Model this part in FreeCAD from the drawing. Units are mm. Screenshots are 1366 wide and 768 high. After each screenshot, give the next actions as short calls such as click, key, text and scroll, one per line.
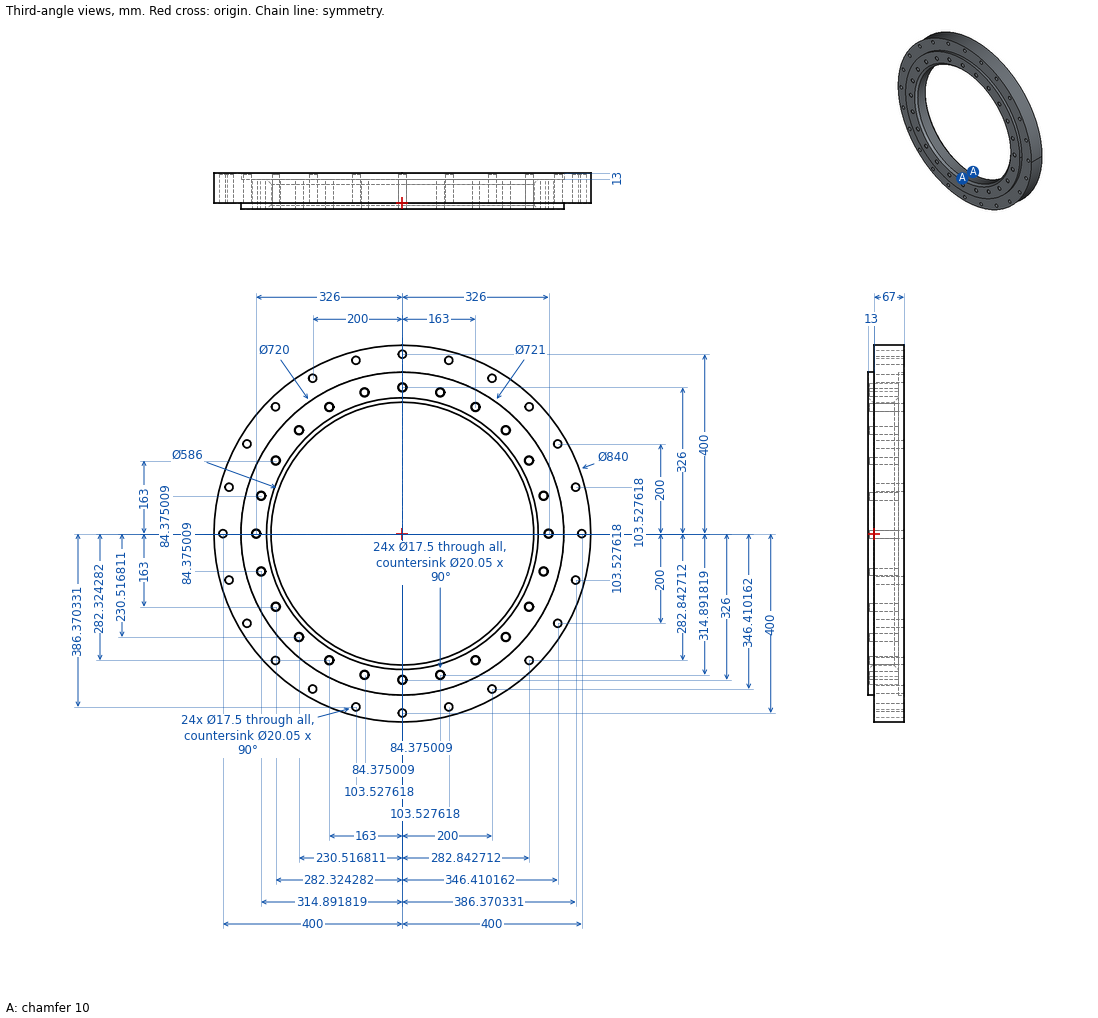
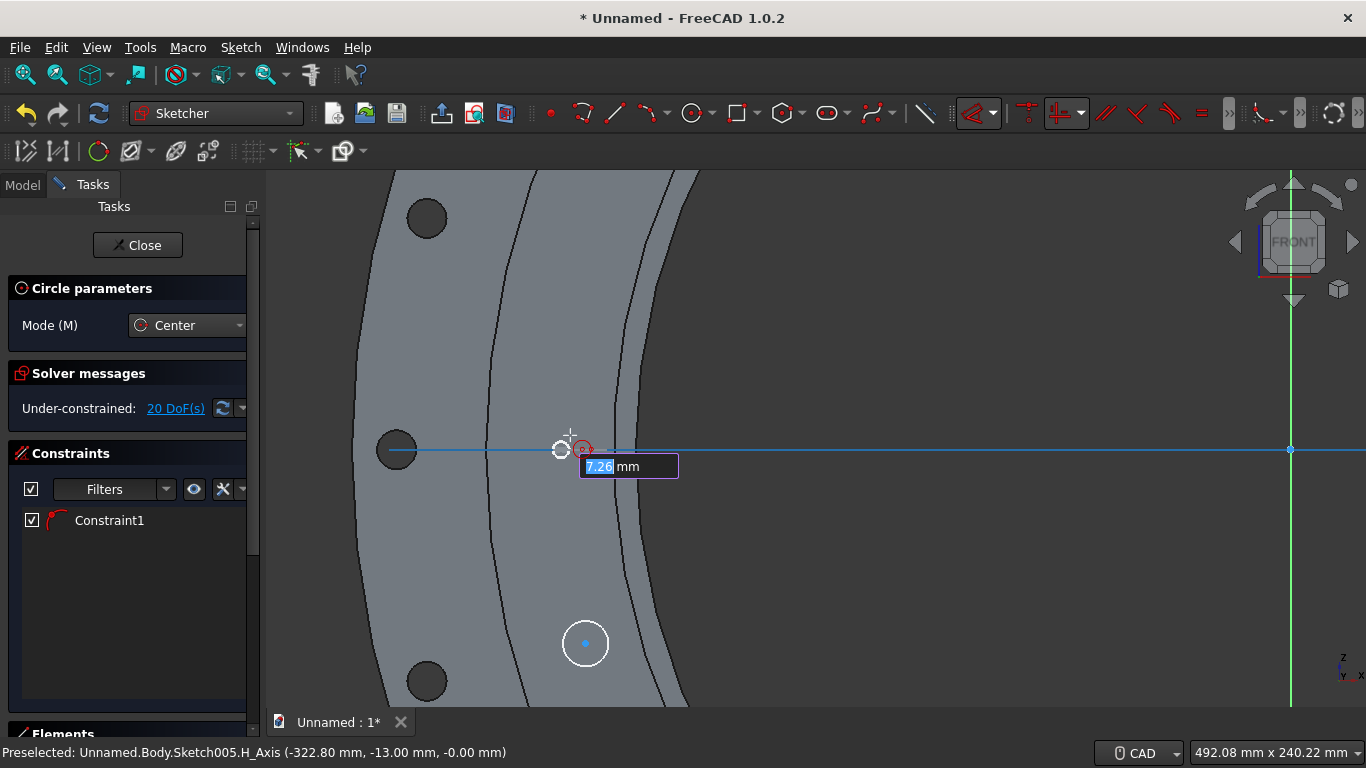
click(569, 431)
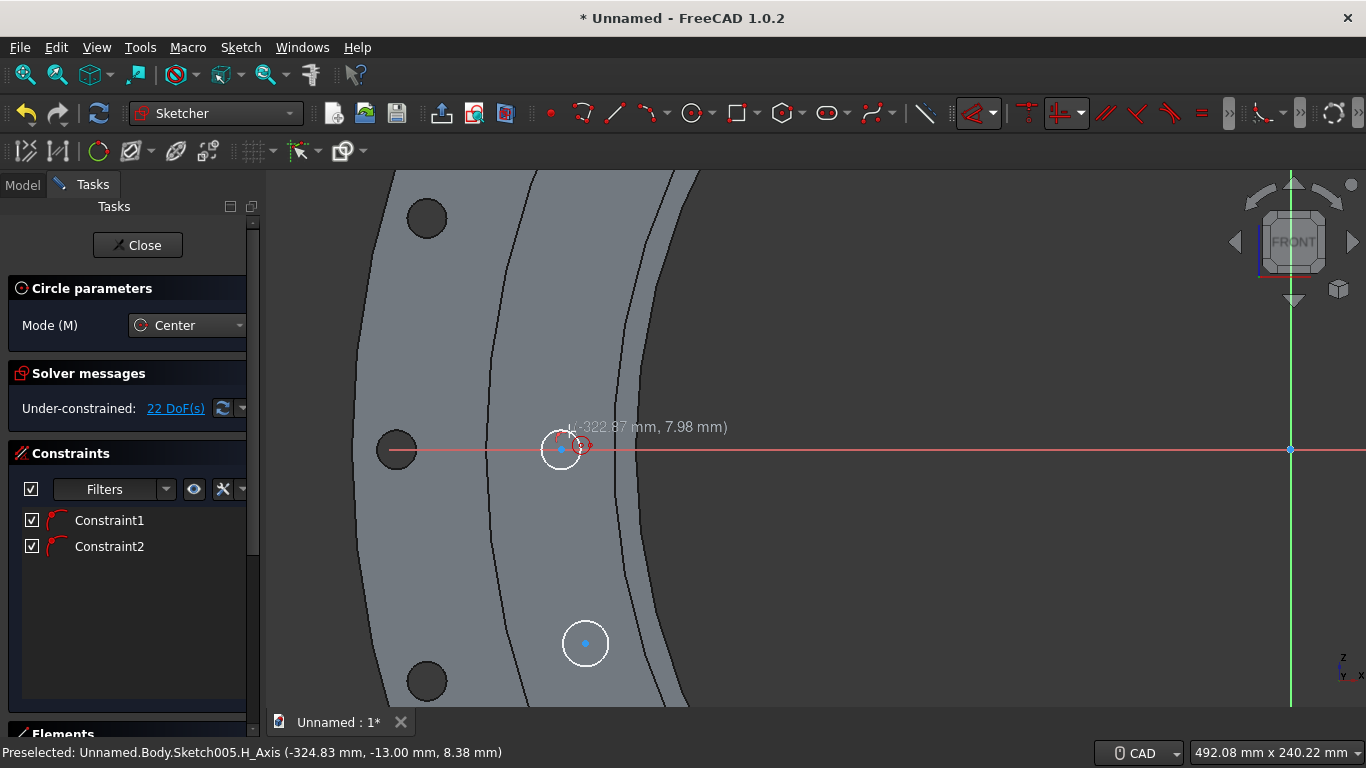
scroll(570, 435, down, 7)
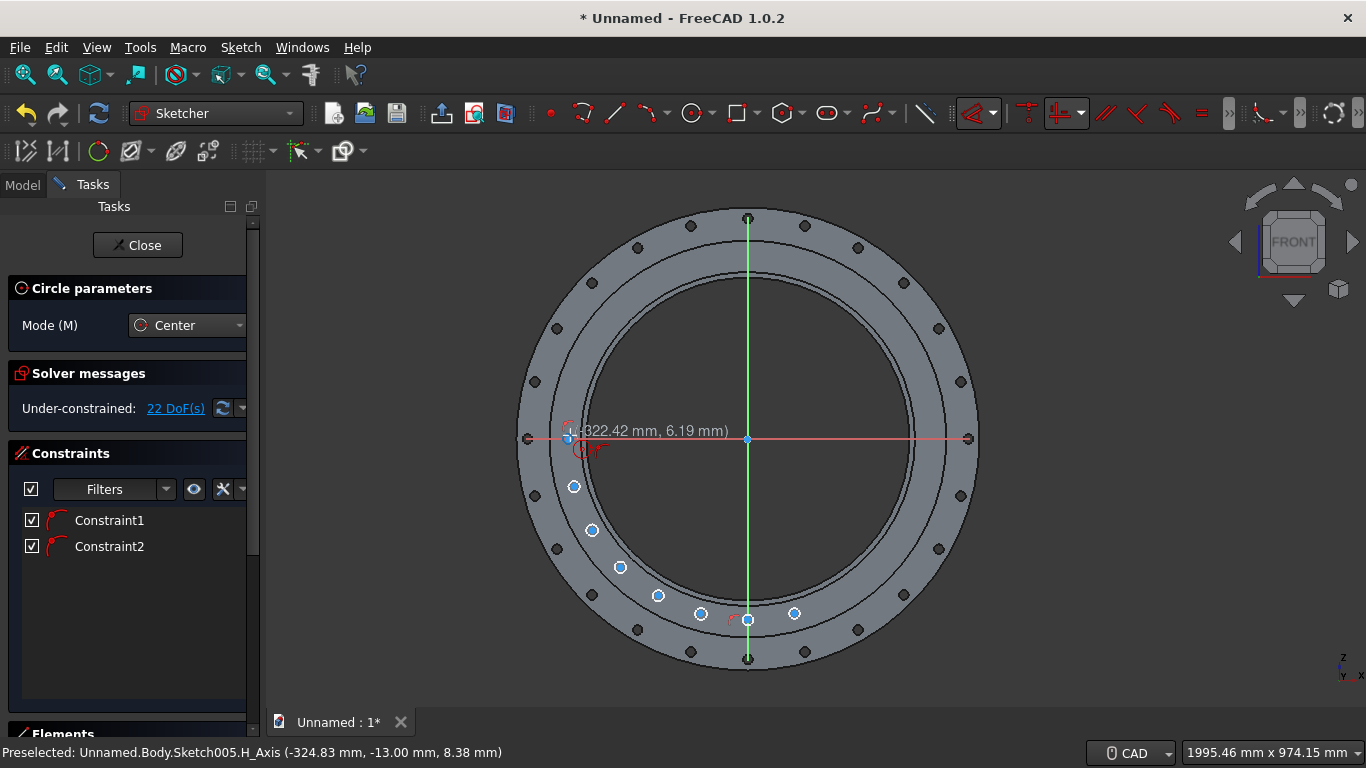
click(574, 393)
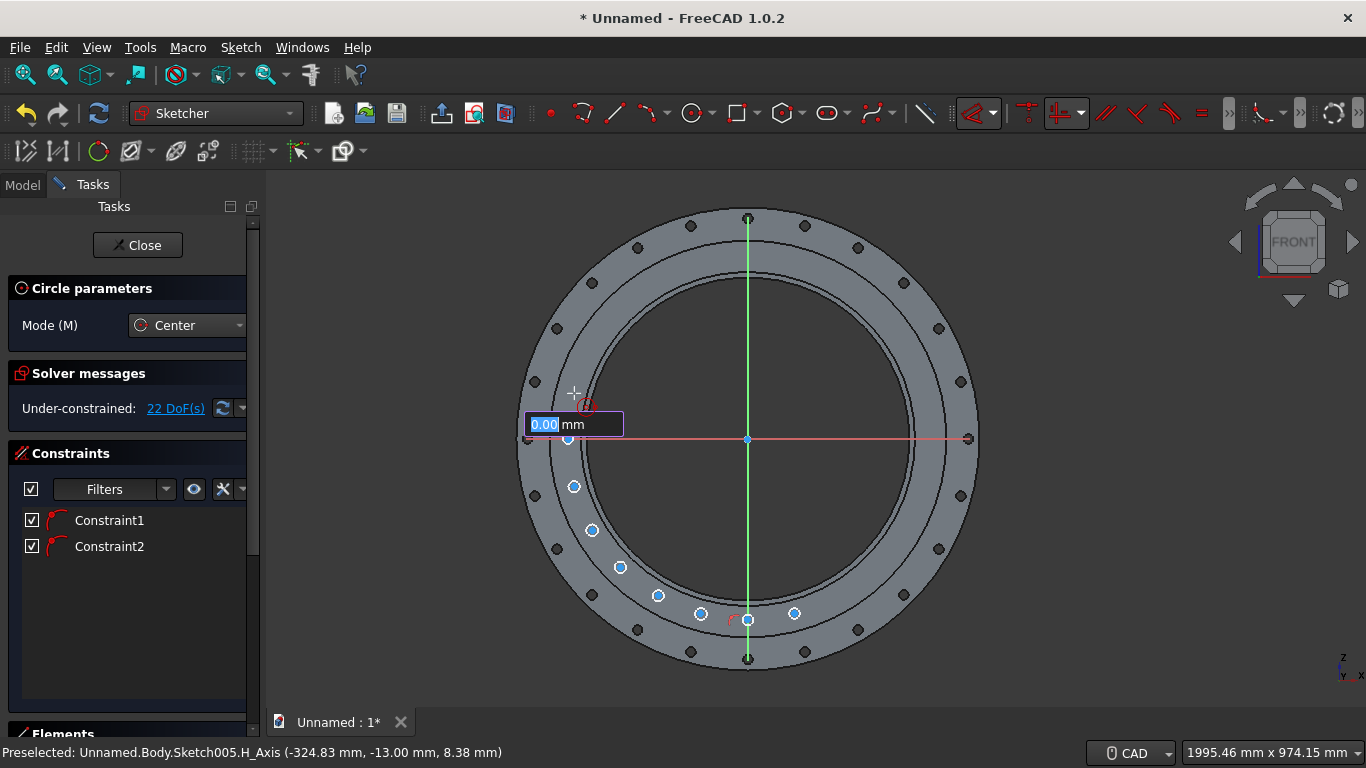
scroll(578, 389, up, 6)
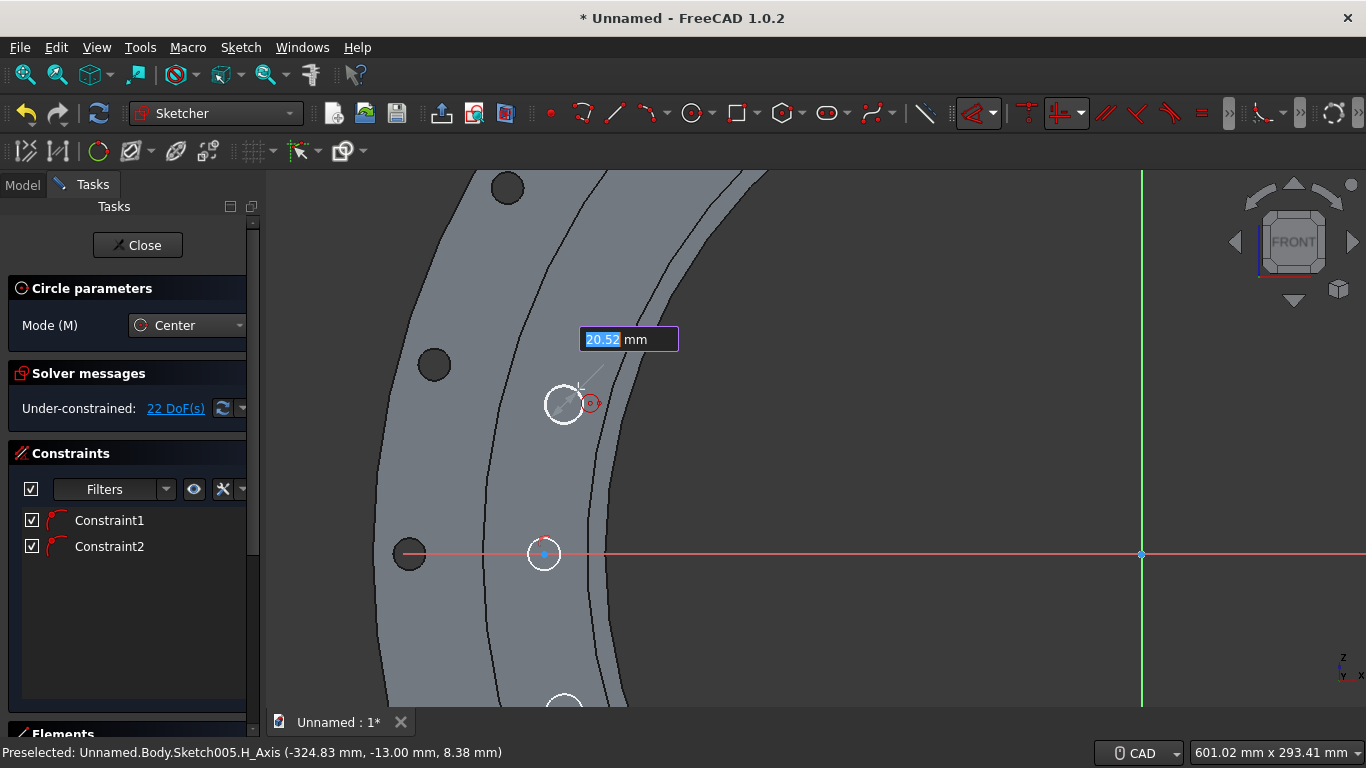
click(577, 388)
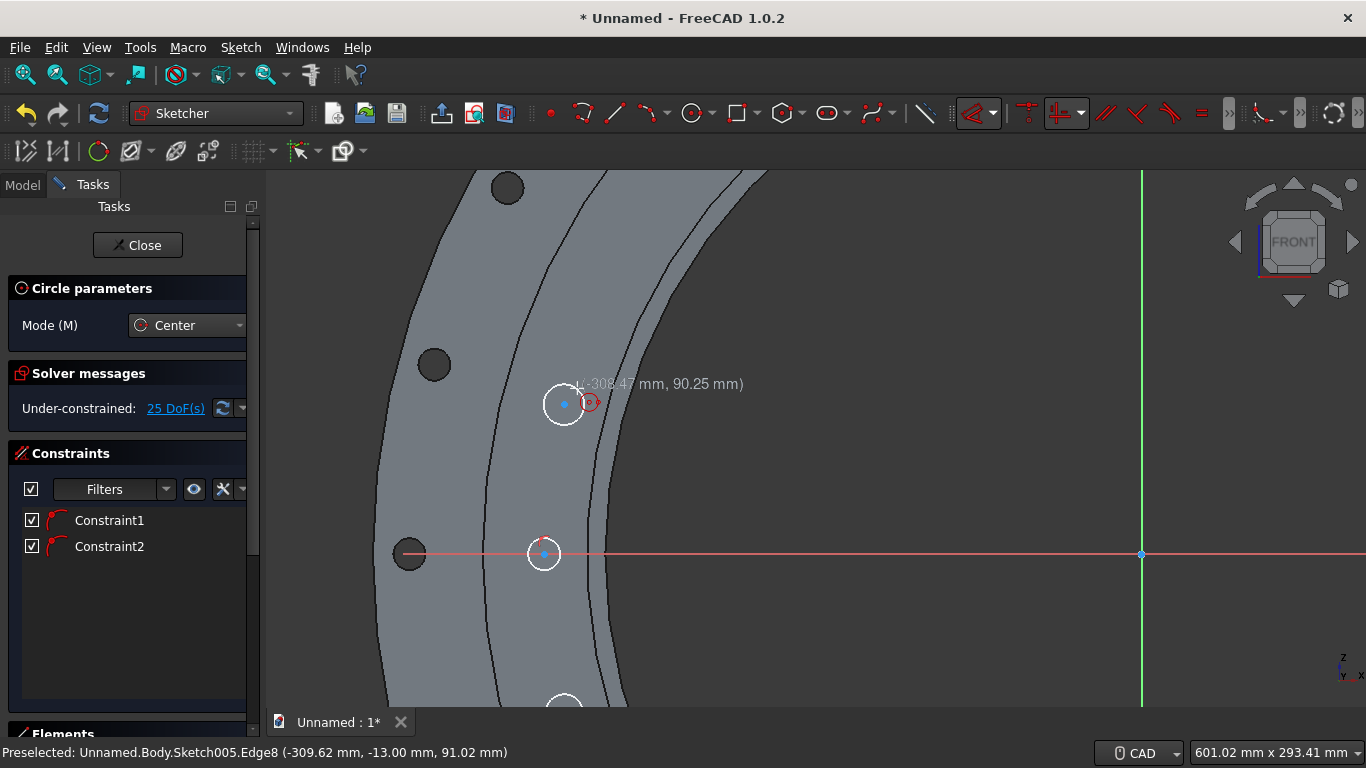
scroll(625, 256, up, 2)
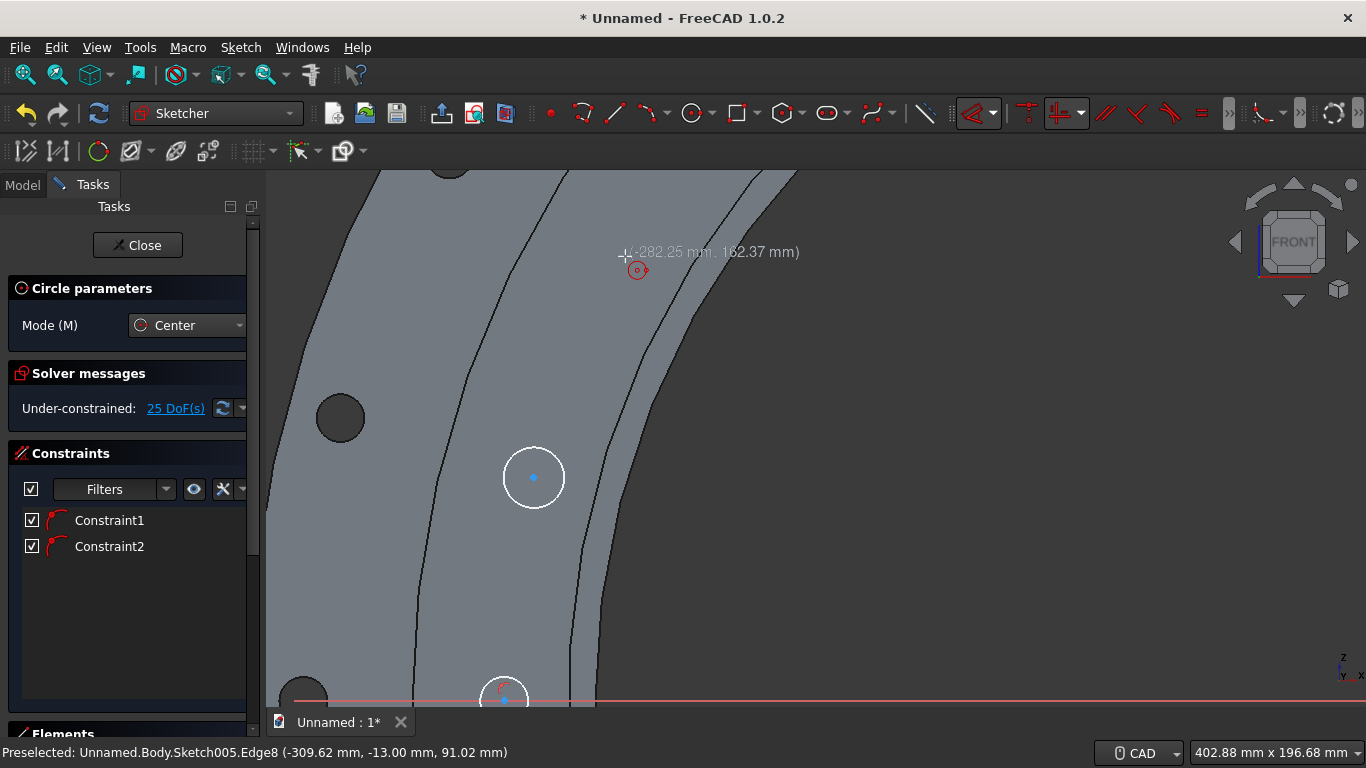
scroll(584, 372, down, 8)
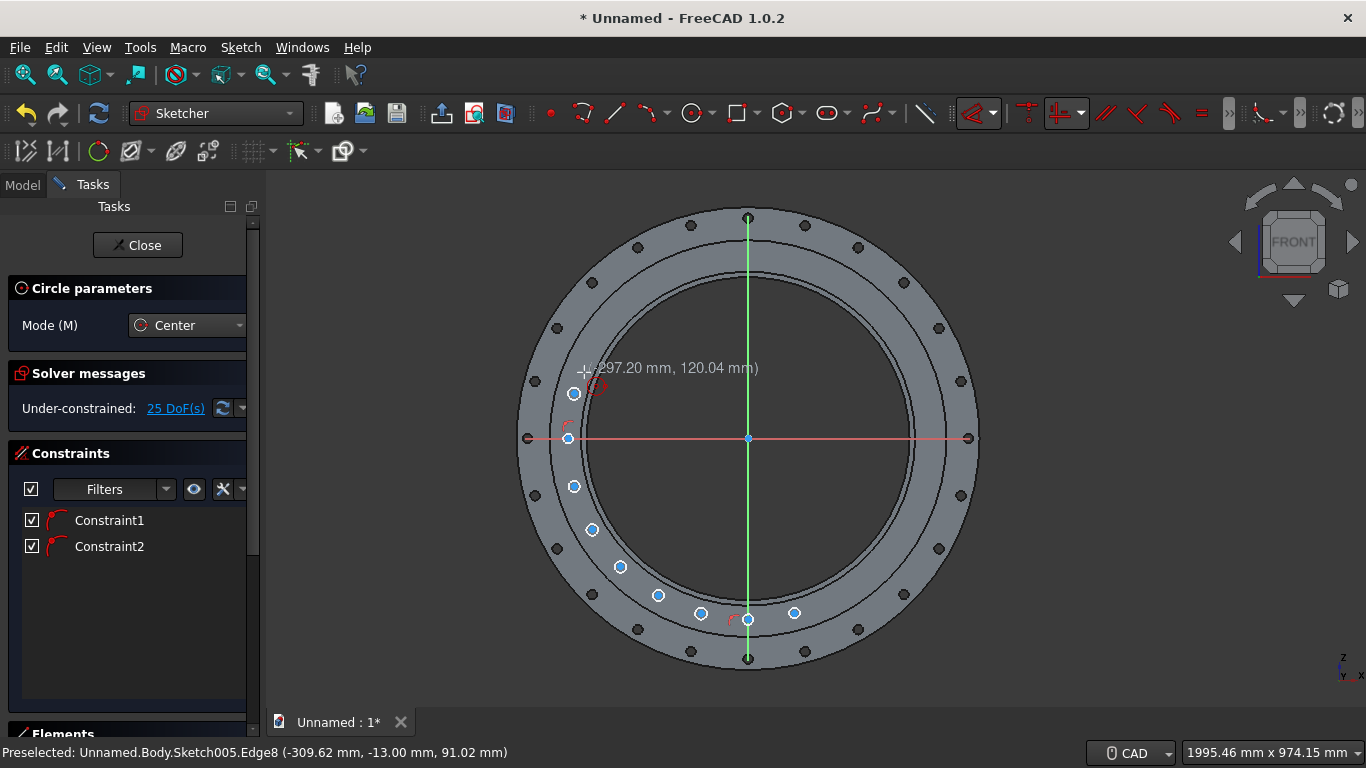
click(592, 349)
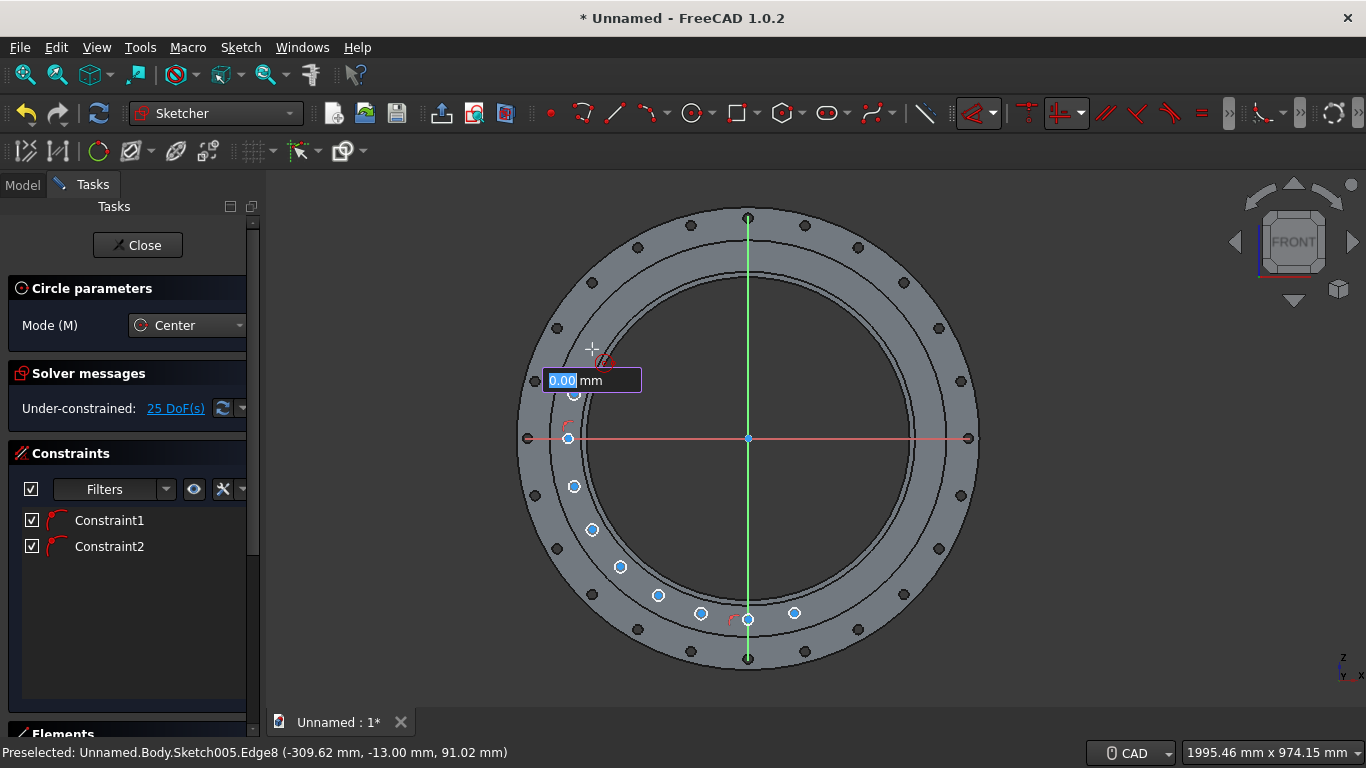
scroll(596, 345, up, 6)